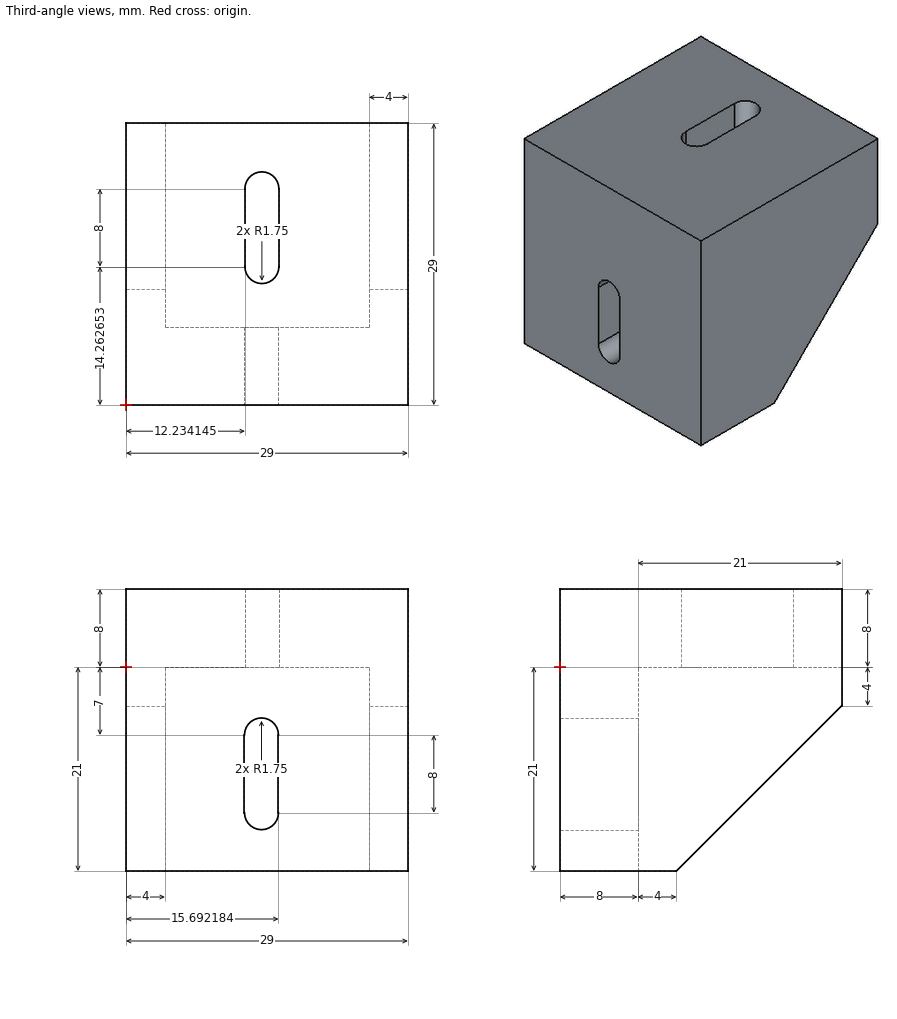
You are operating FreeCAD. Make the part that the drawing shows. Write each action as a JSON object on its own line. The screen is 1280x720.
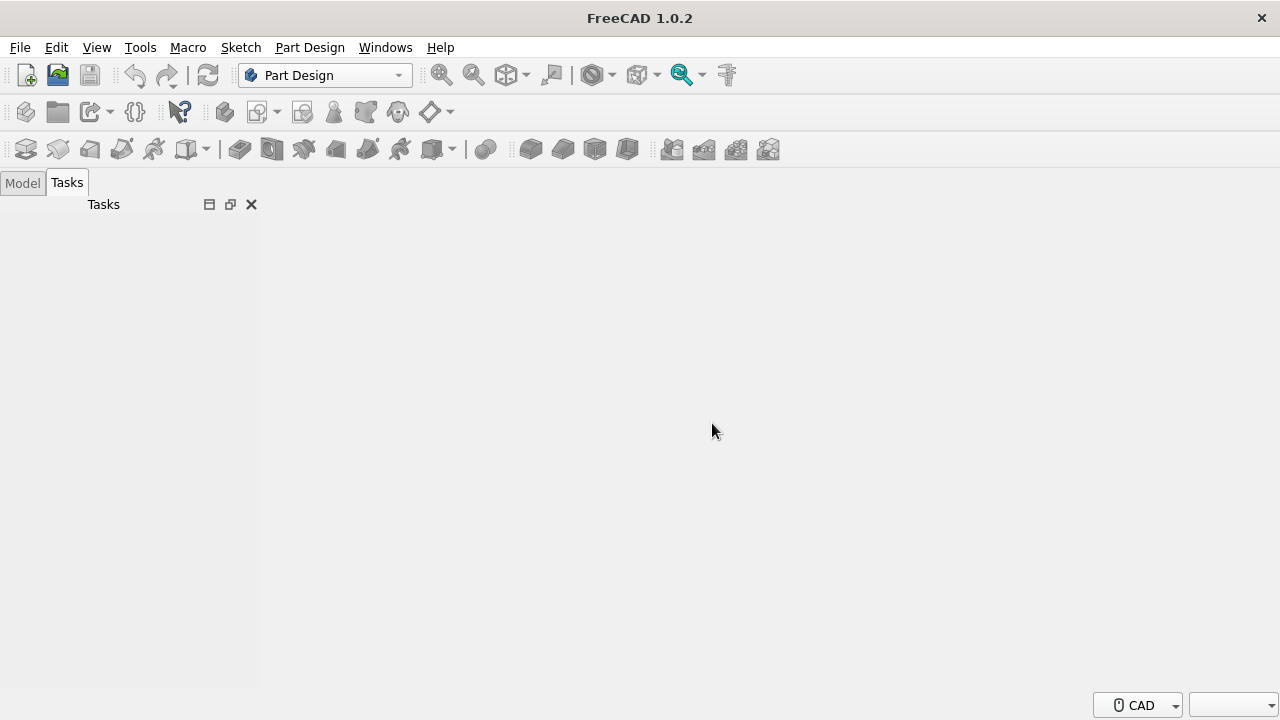
{"action": "left_click", "coordinate": [26, 76]}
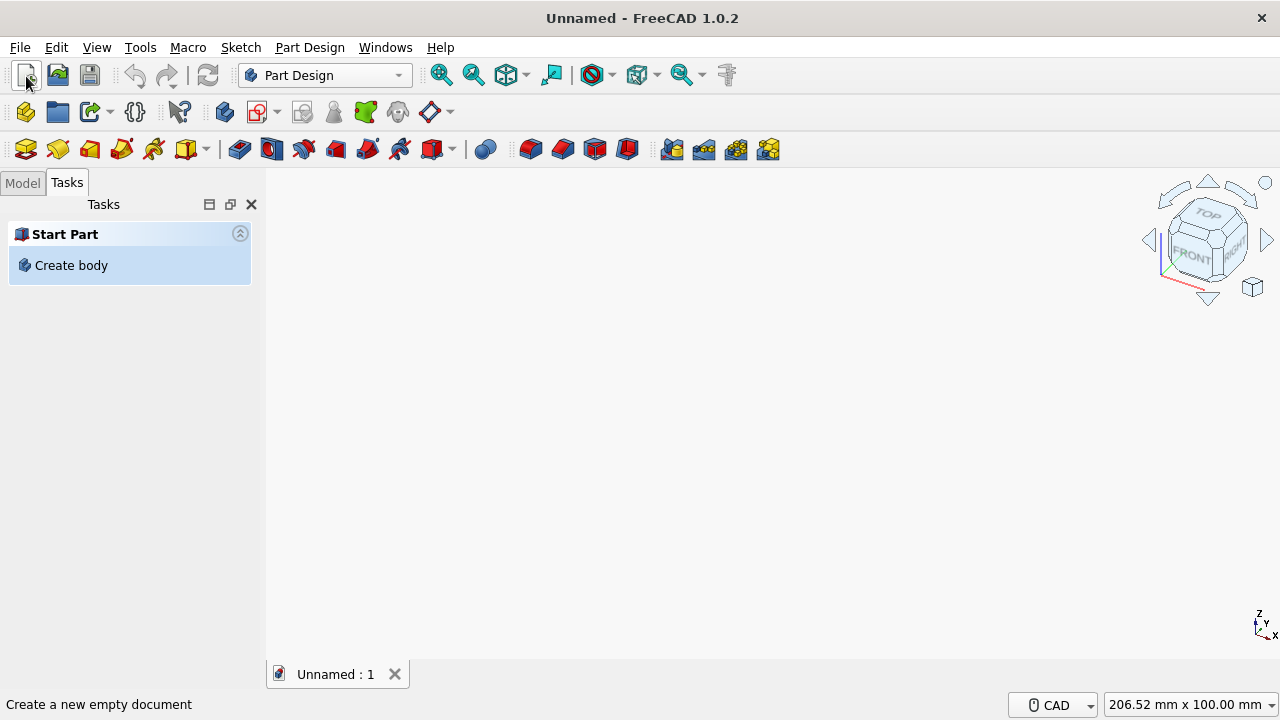
{"action": "left_click", "coordinate": [258, 112]}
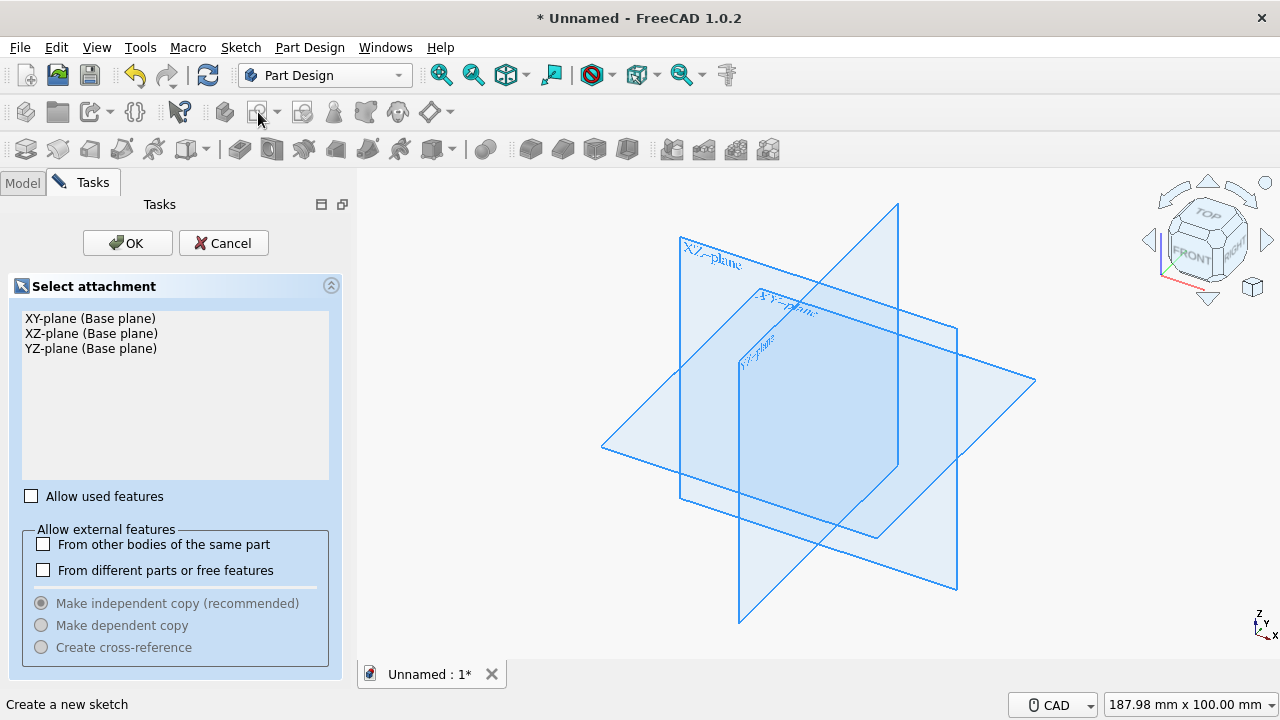
{"action": "left_click", "coordinate": [82, 318]}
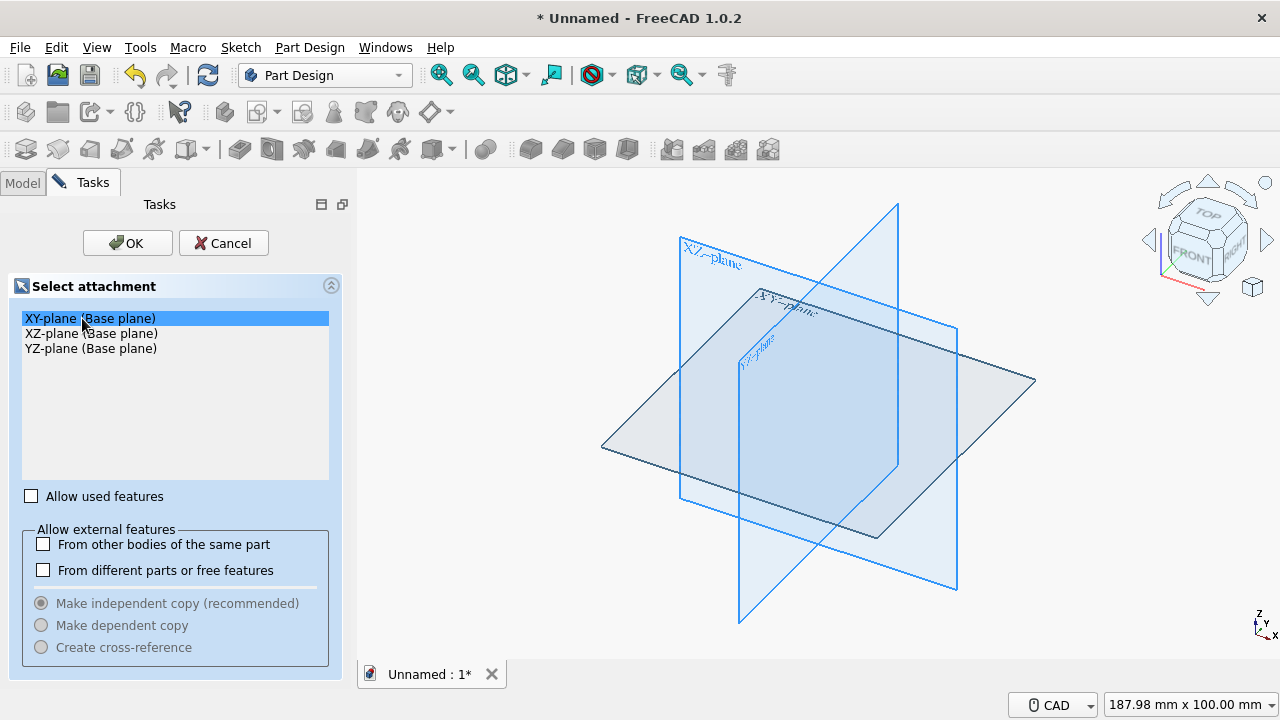
{"action": "left_click", "coordinate": [128, 243]}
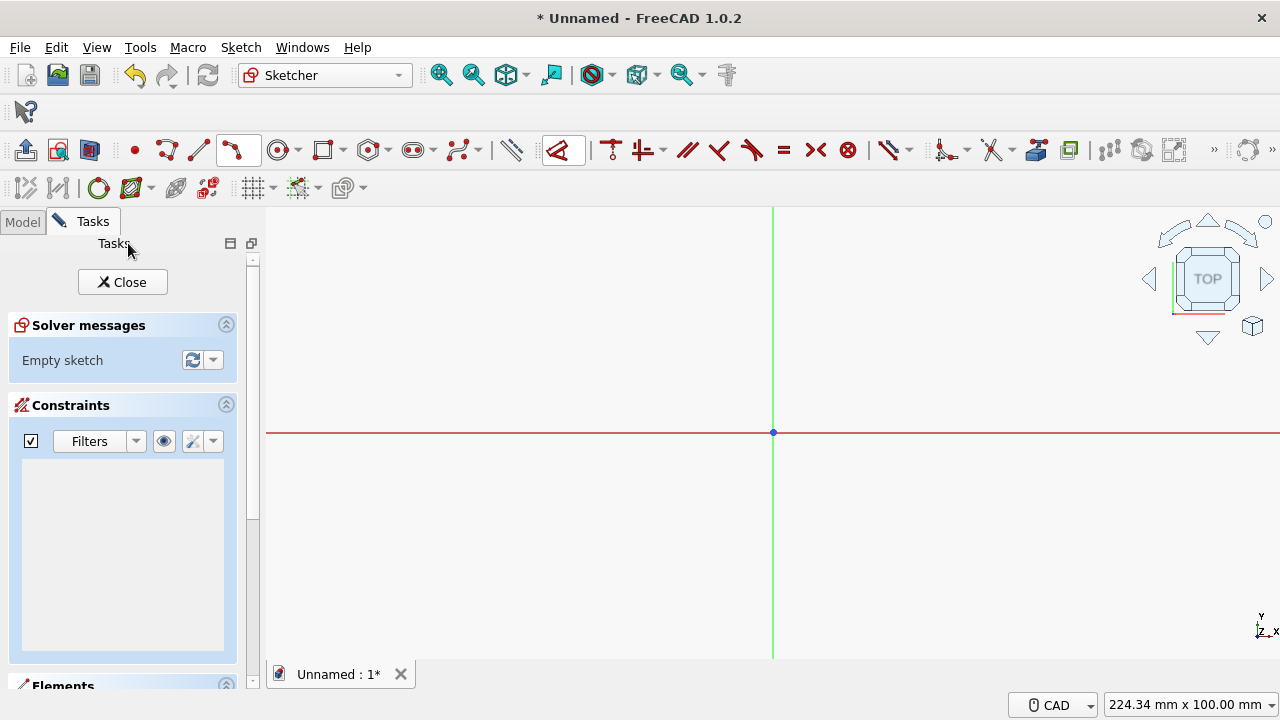
{"action": "scroll", "coordinate": [948, 314], "scroll_direction": "up", "scroll_amount": 4}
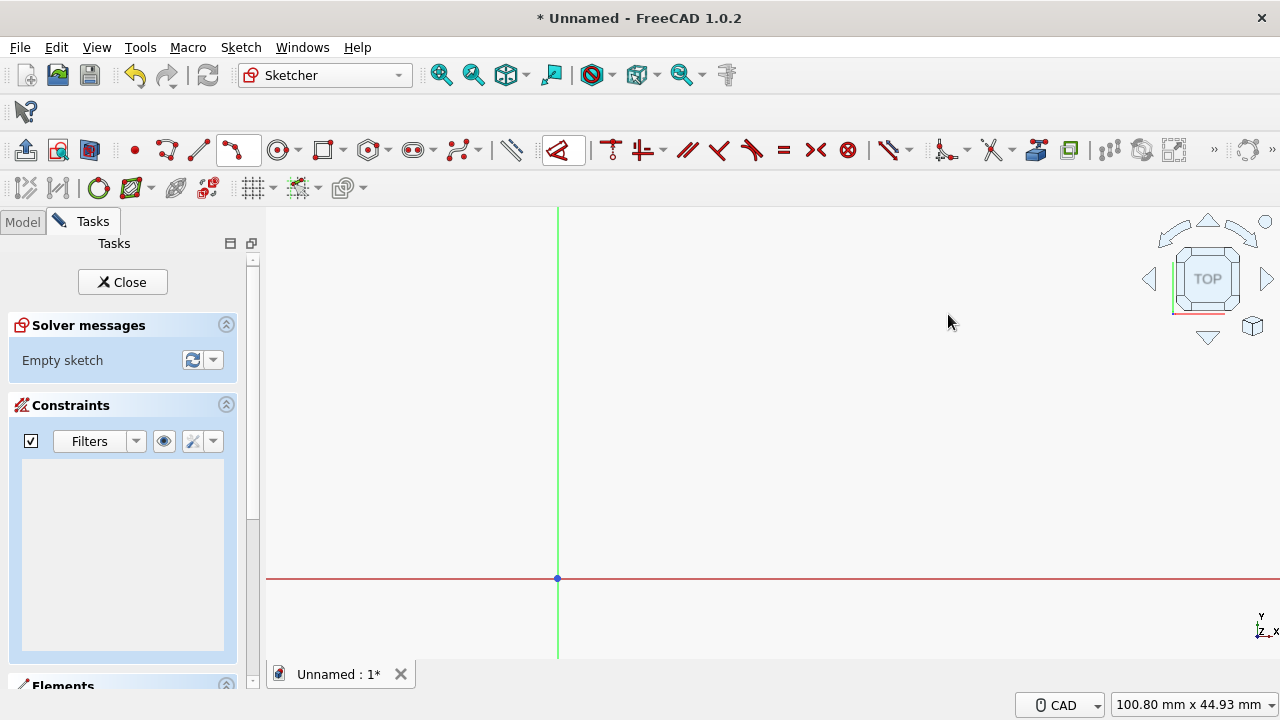
{"action": "key", "text": "g r"}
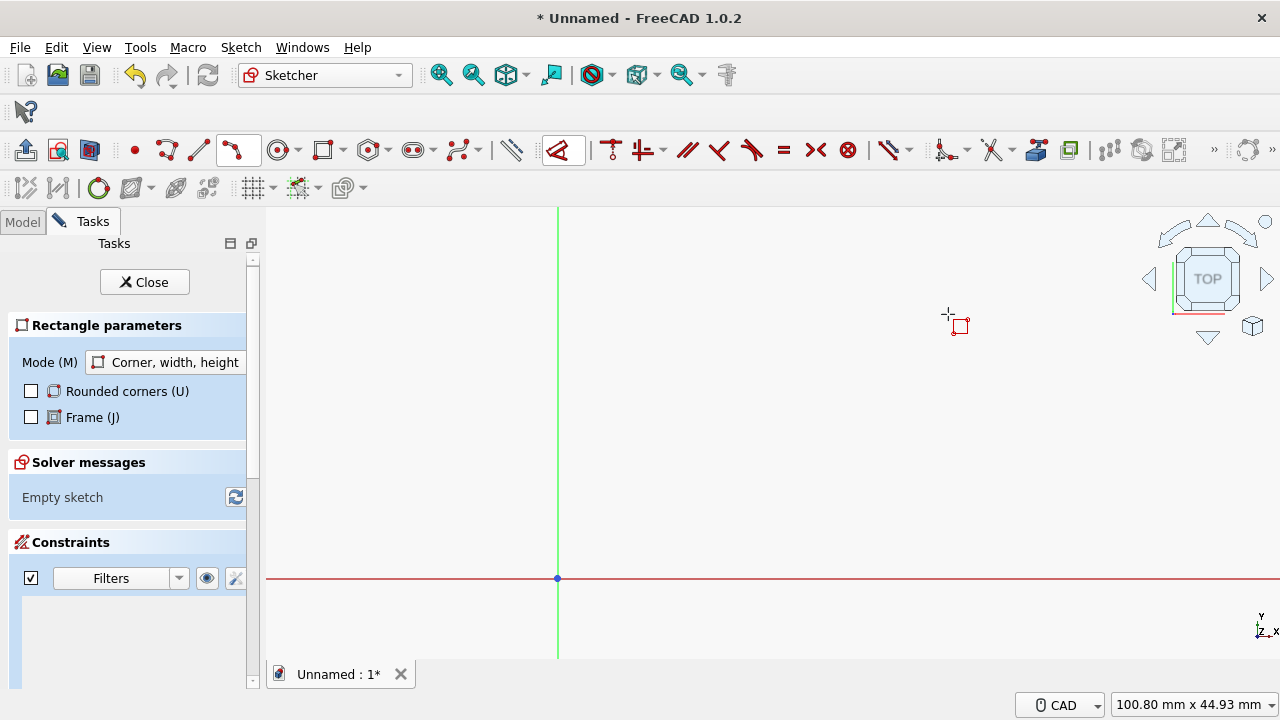
{"action": "left_click", "coordinate": [558, 579]}
{"action": "left_click", "coordinate": [849, 287]}
{"action": "key", "text": "Escape"}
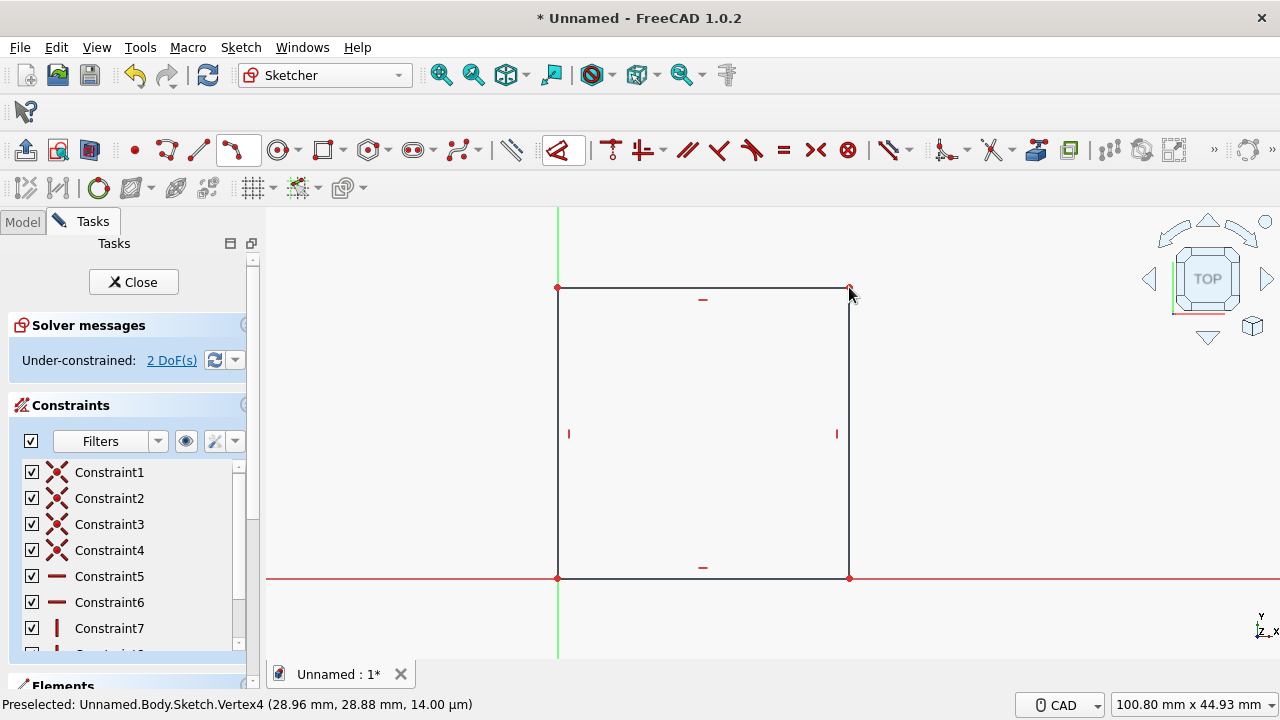
{"action": "left_click", "coordinate": [645, 579]}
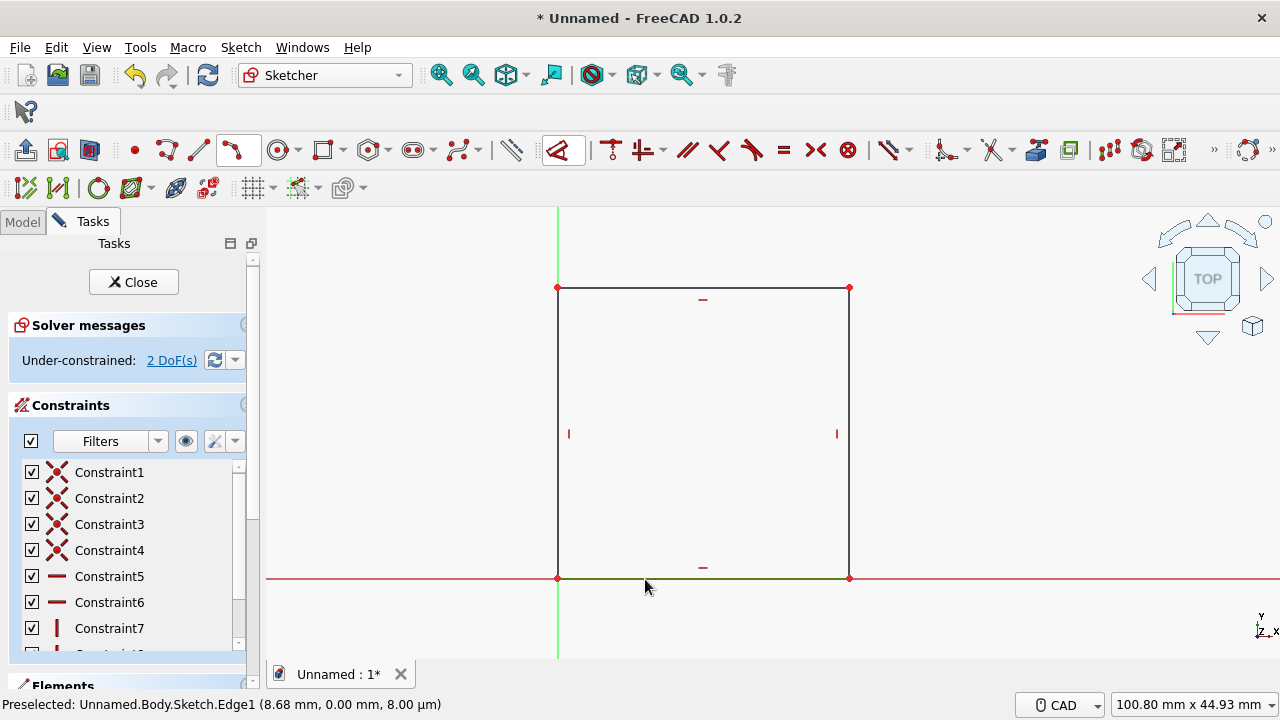
{"action": "key", "text": "l"}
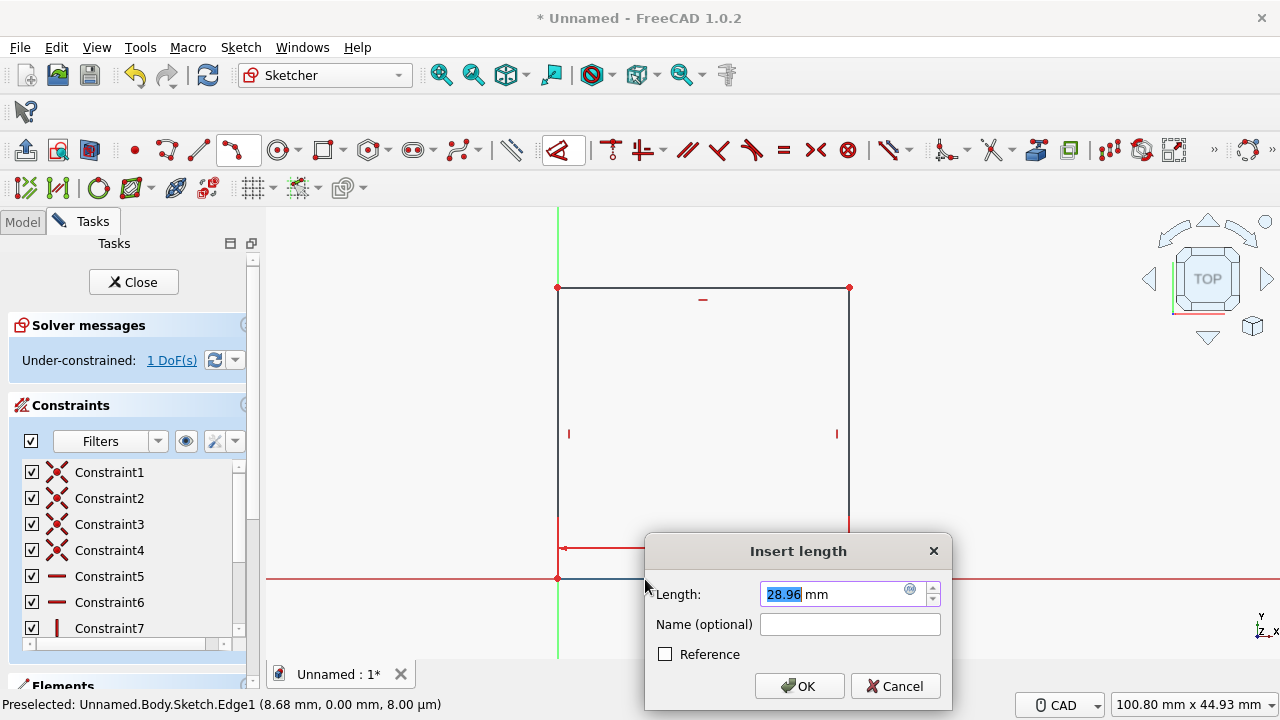
{"action": "type", "text": "29"}
{"action": "key", "text": "Return"}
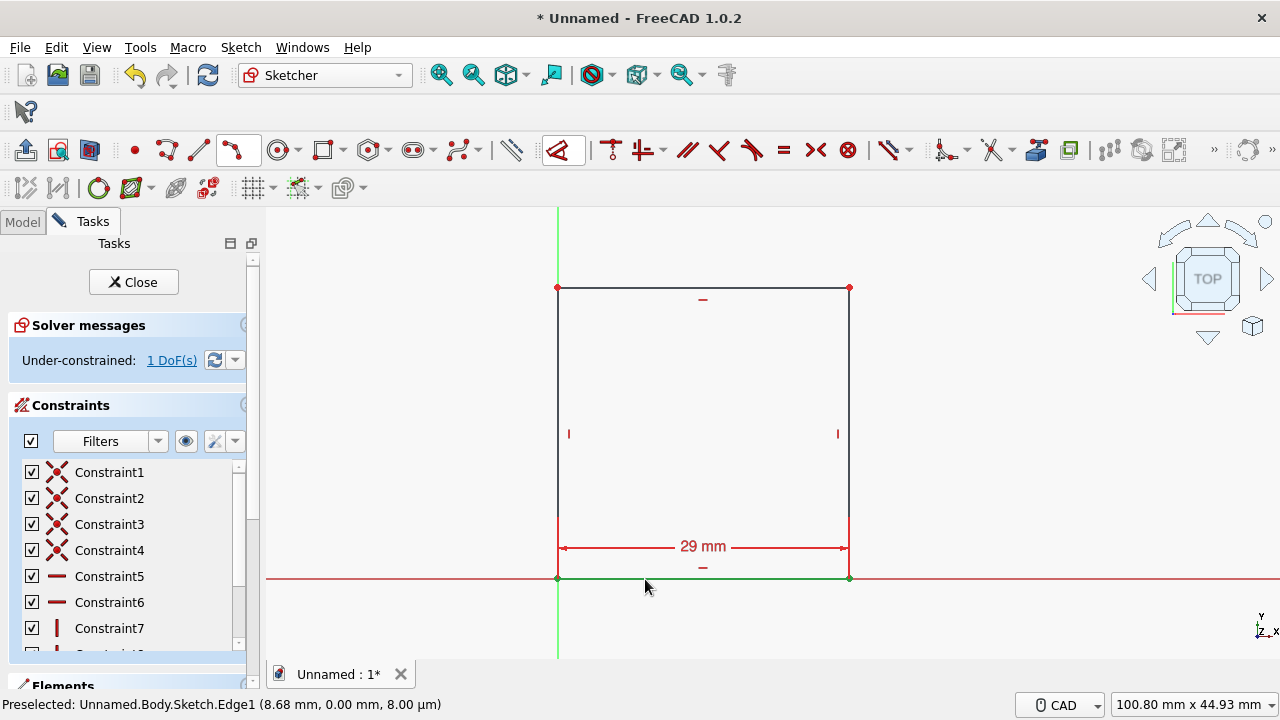
{"action": "left_click", "coordinate": [849, 491]}